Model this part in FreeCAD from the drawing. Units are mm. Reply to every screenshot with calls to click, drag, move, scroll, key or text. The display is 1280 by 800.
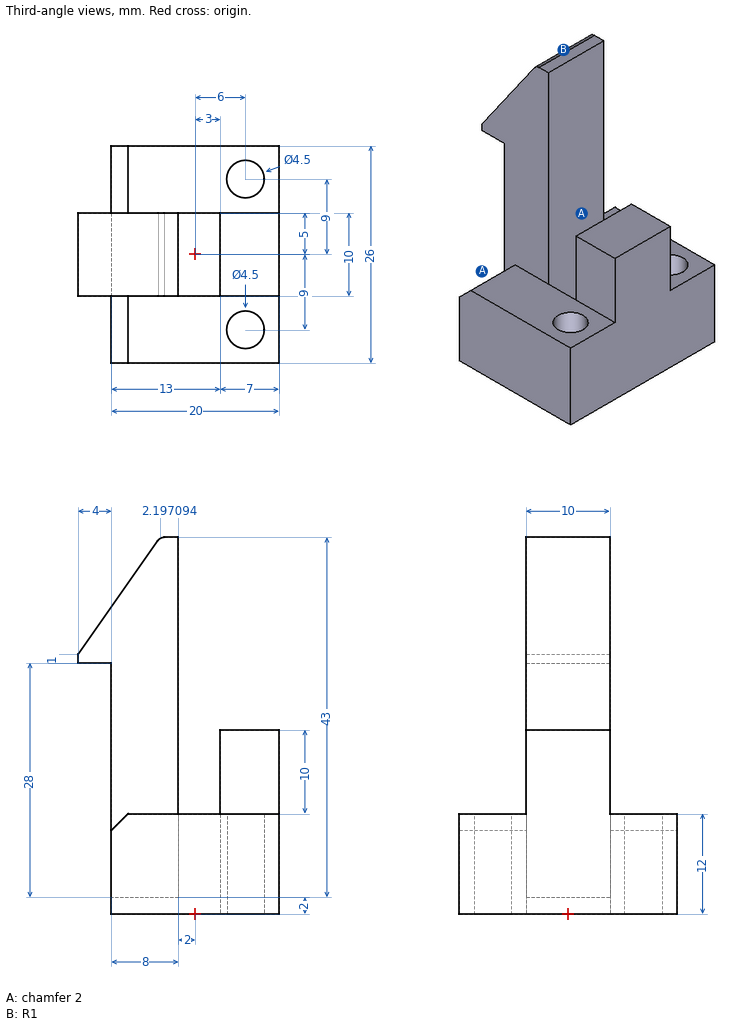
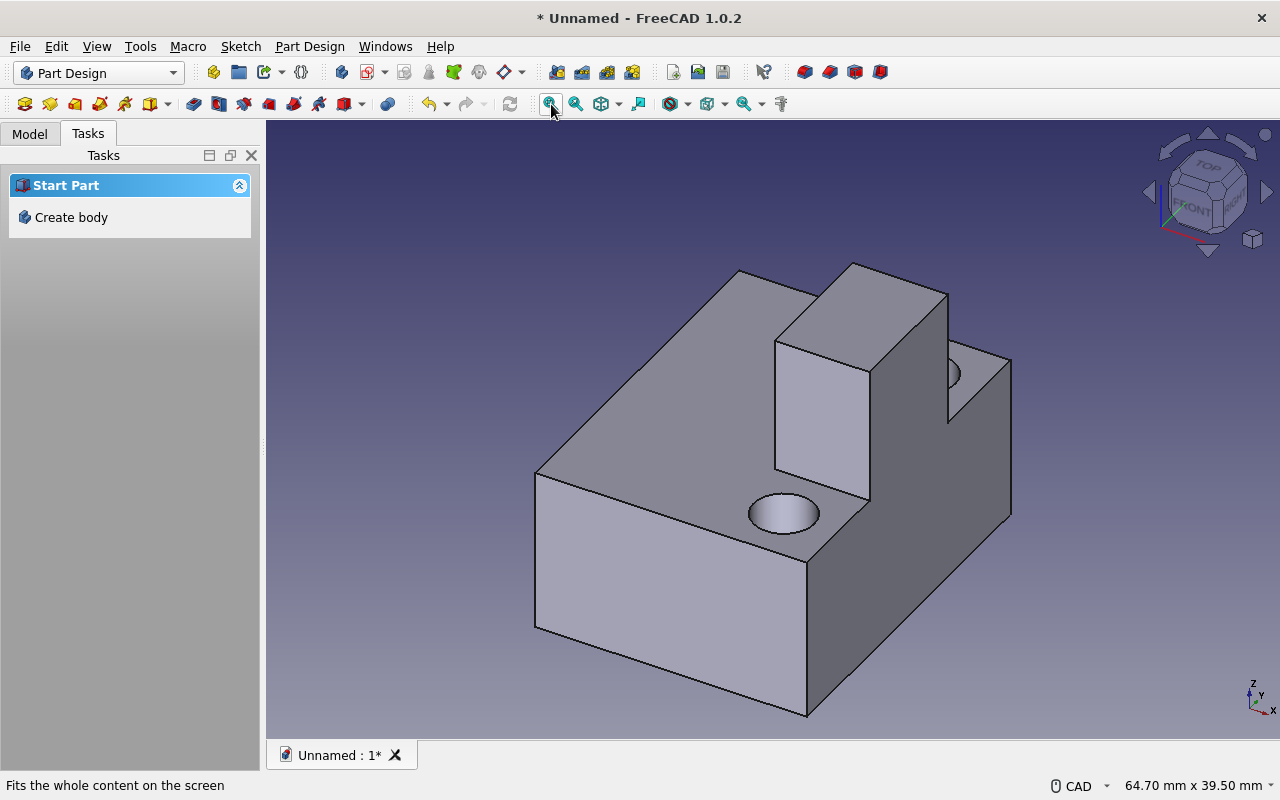
click(763, 374)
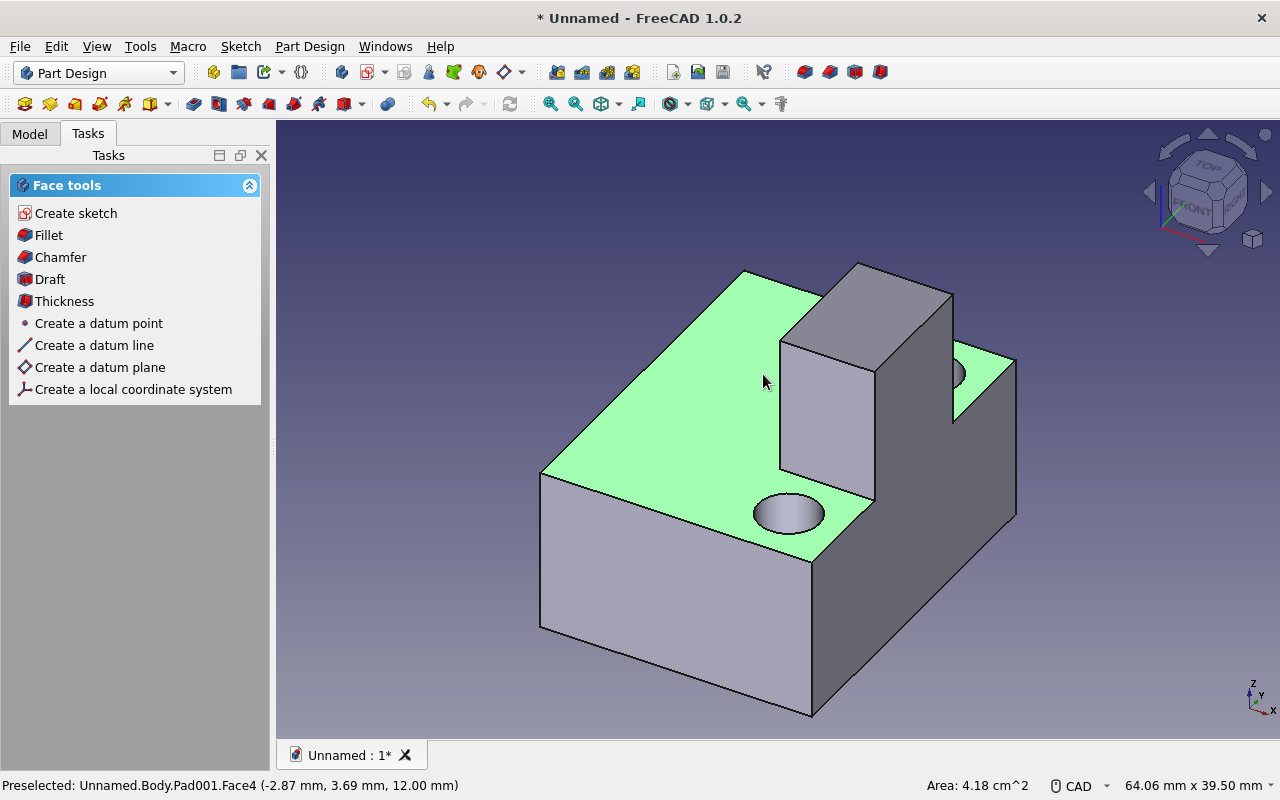
click(366, 72)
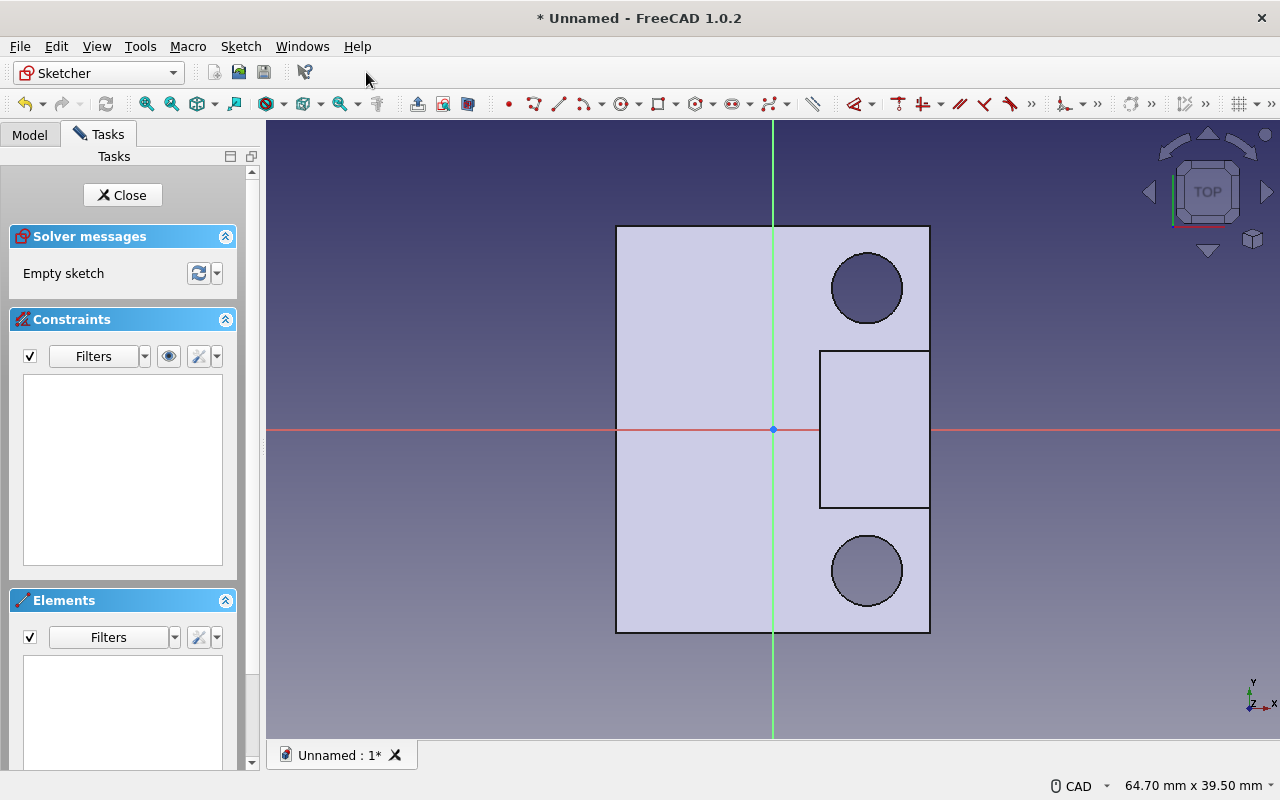
scroll(726, 429, up, 5)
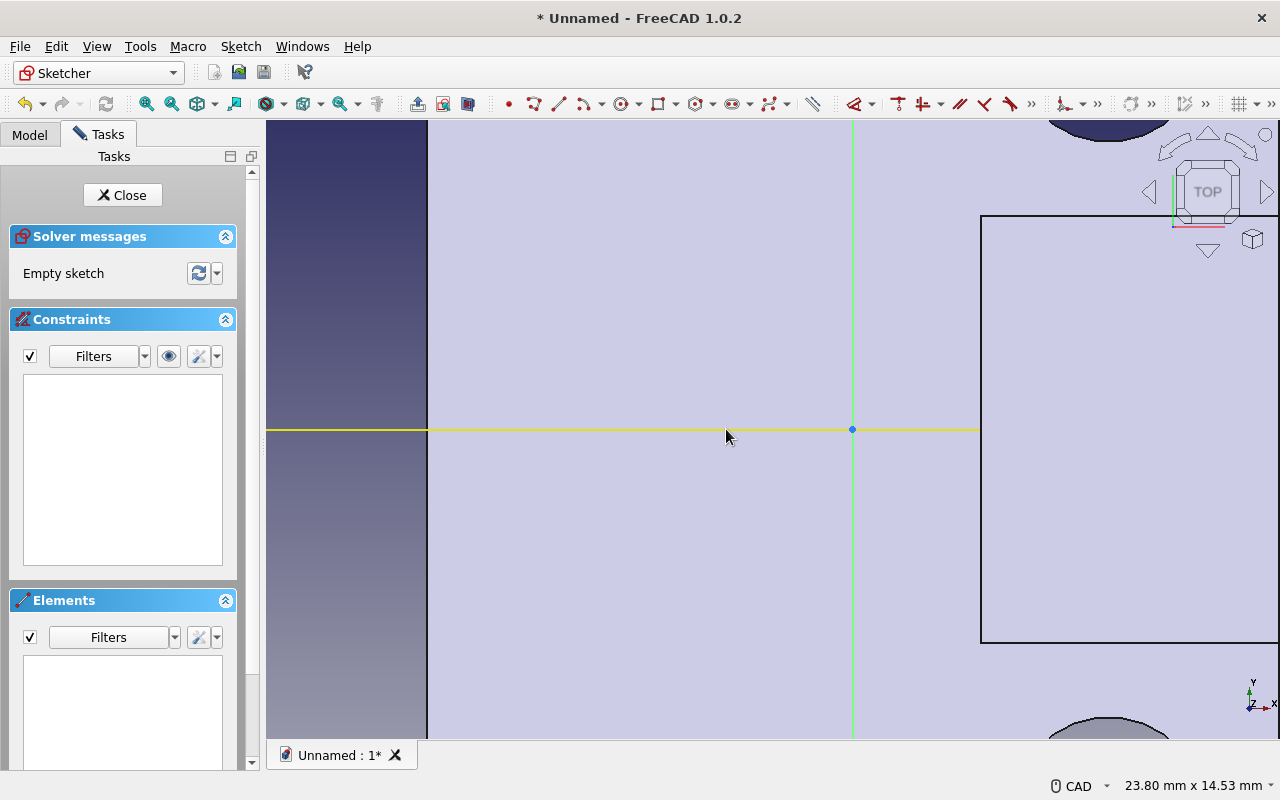
click(658, 104)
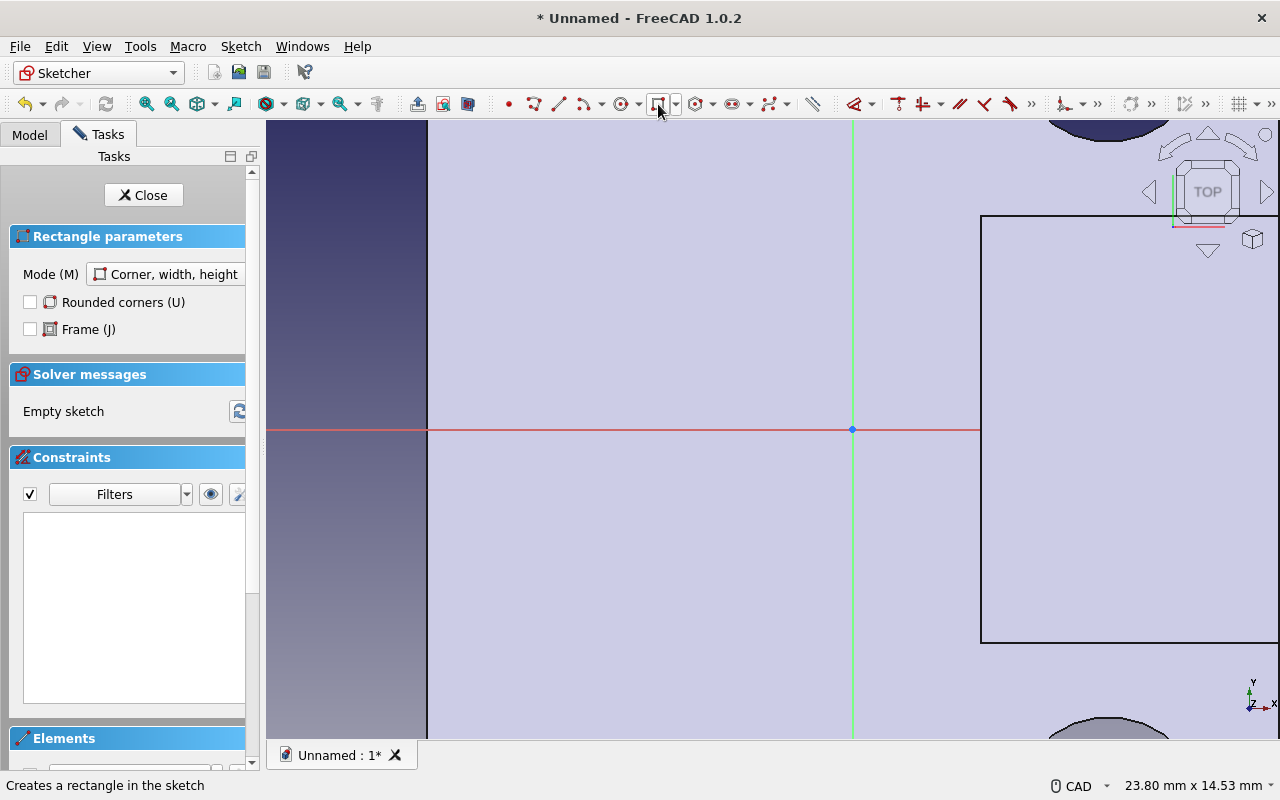
click(427, 216)
click(981, 643)
key(Escape)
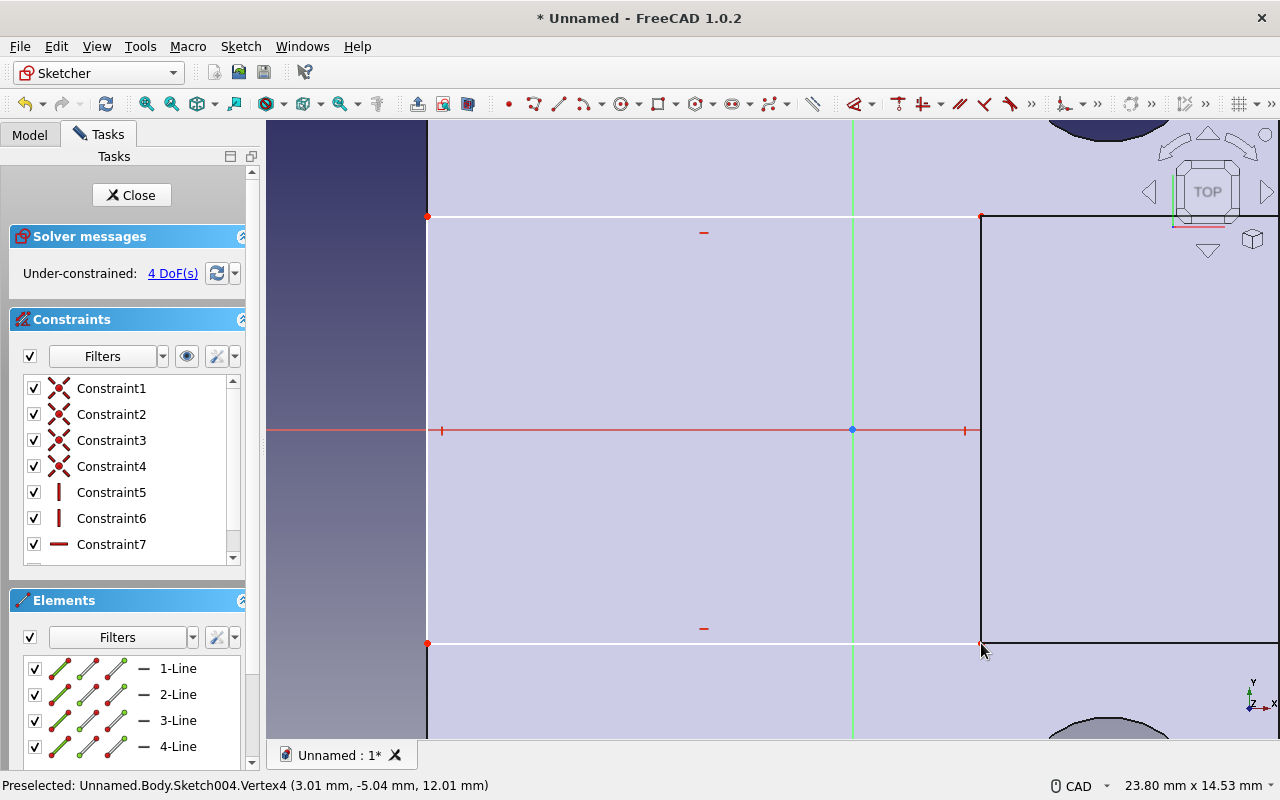
click(854, 104)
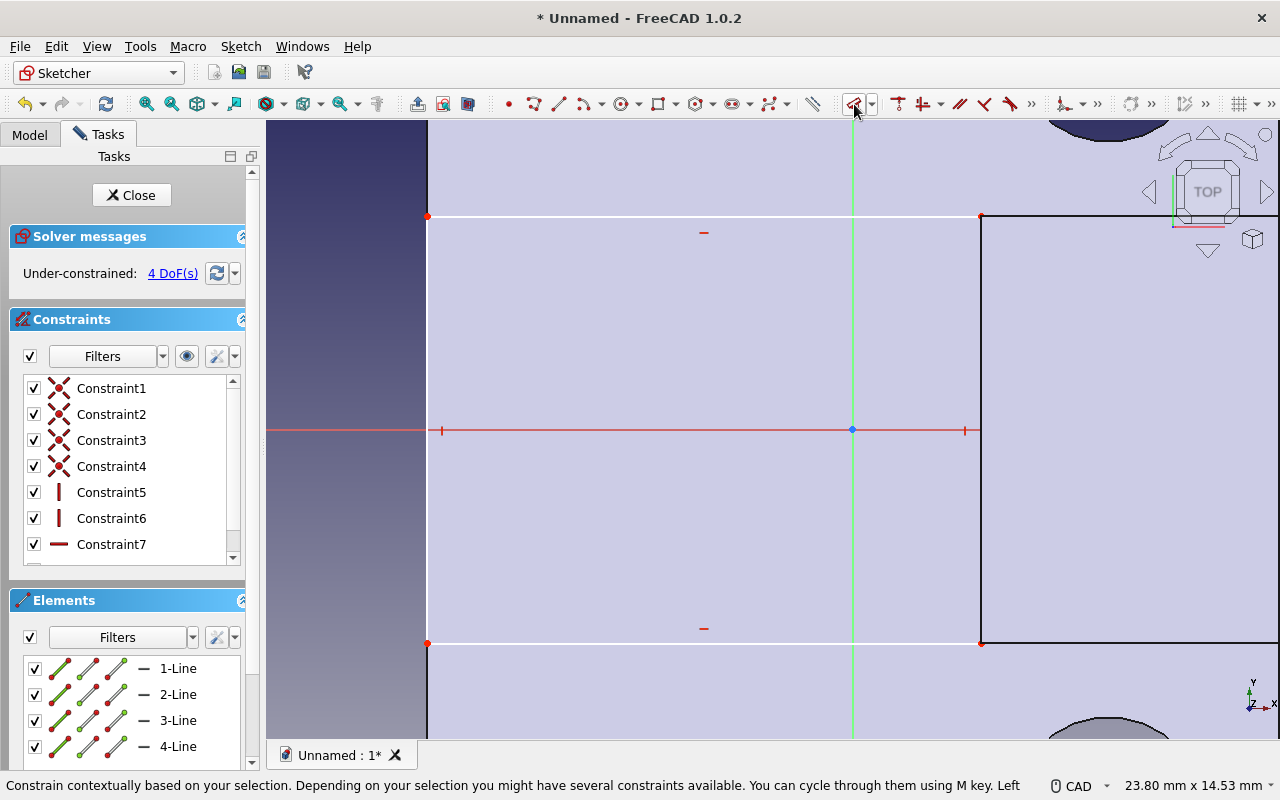
click(427, 345)
click(393, 332)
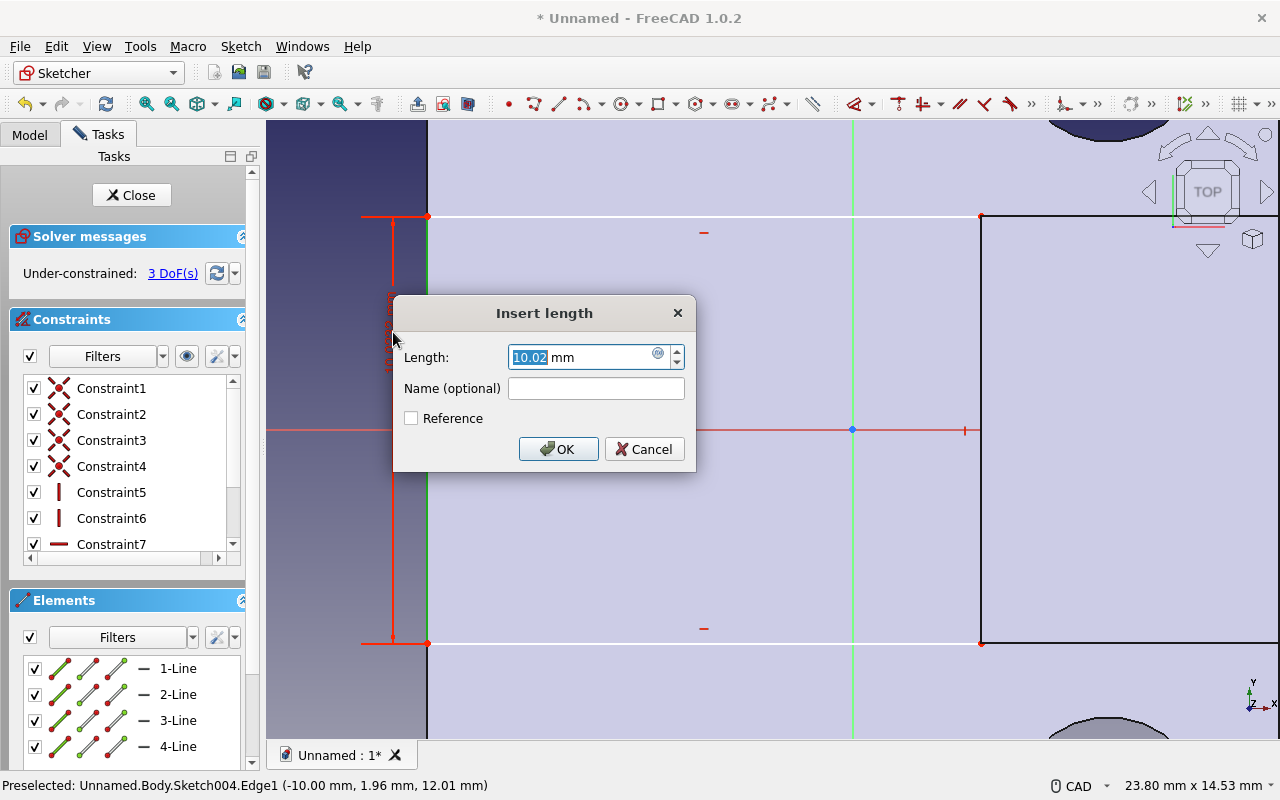
text(10)
key(Return)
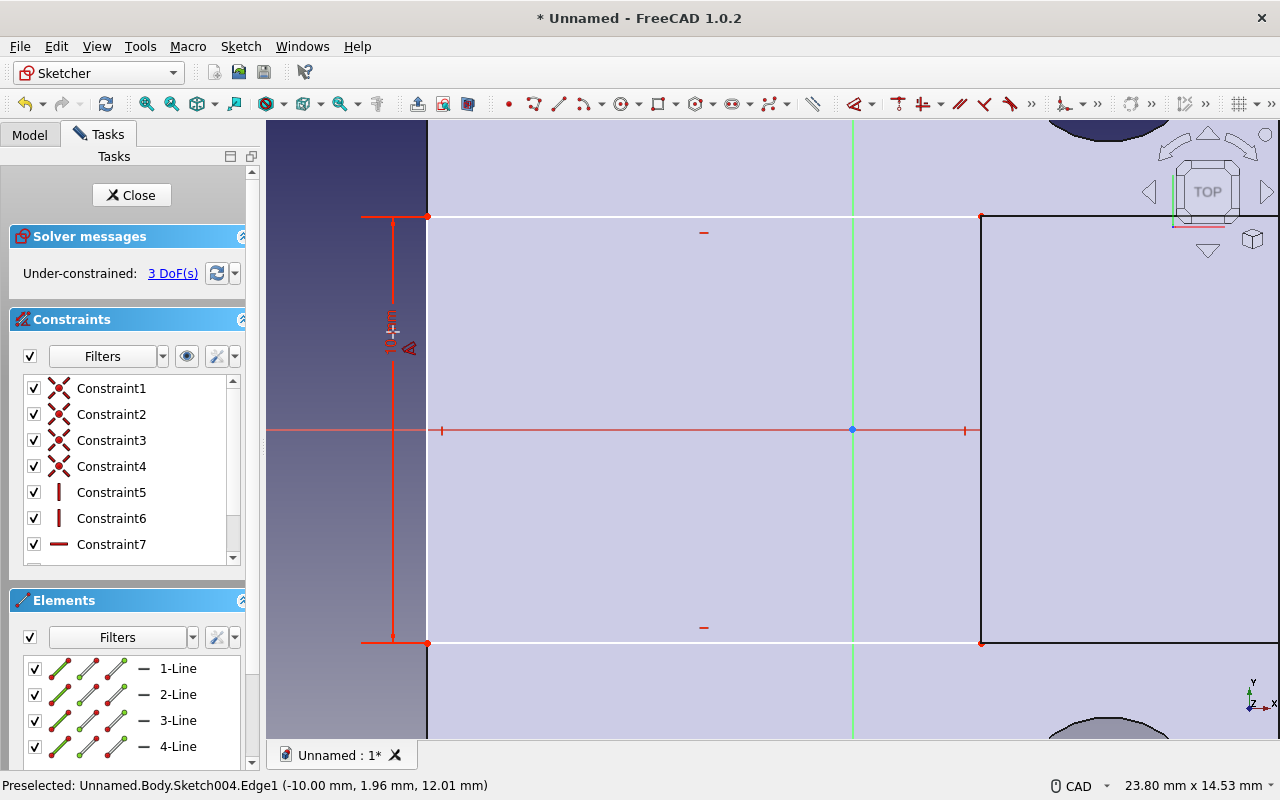
click(593, 643)
click(704, 677)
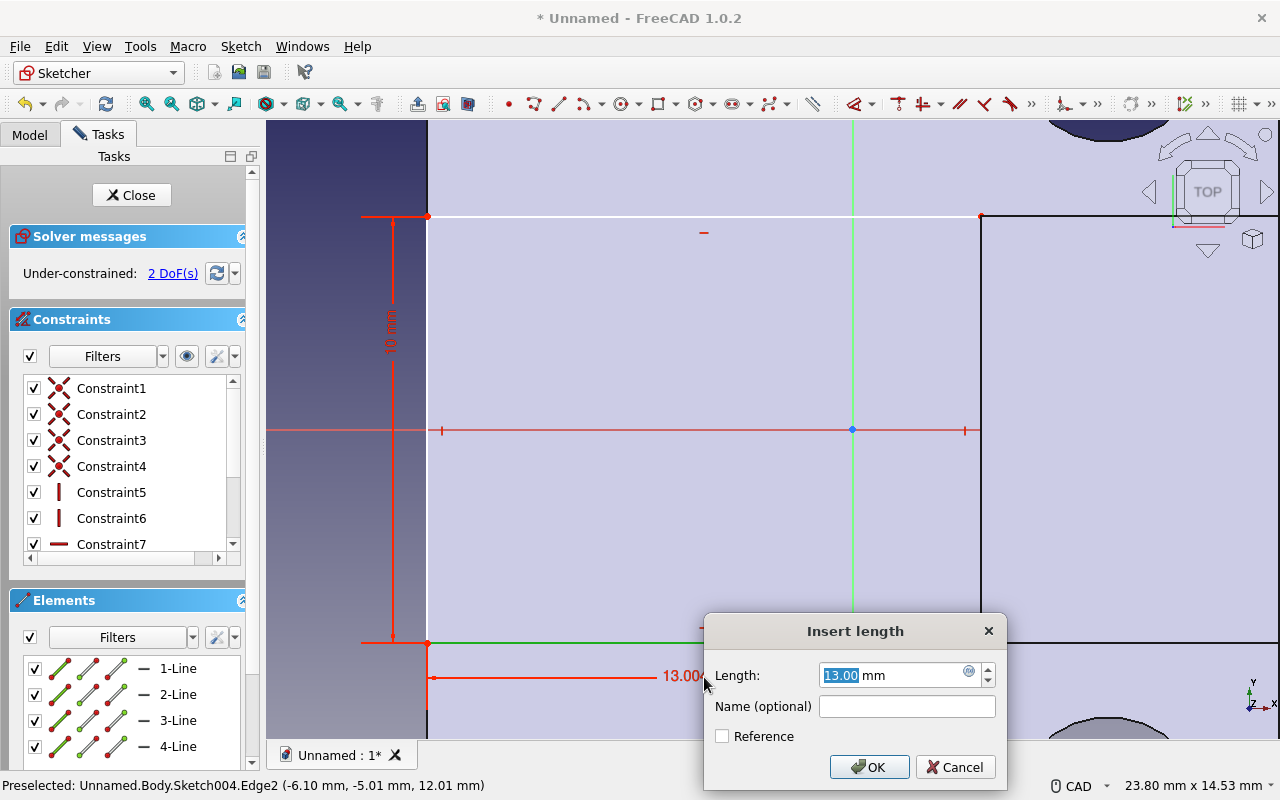
text(13)
key(Return)